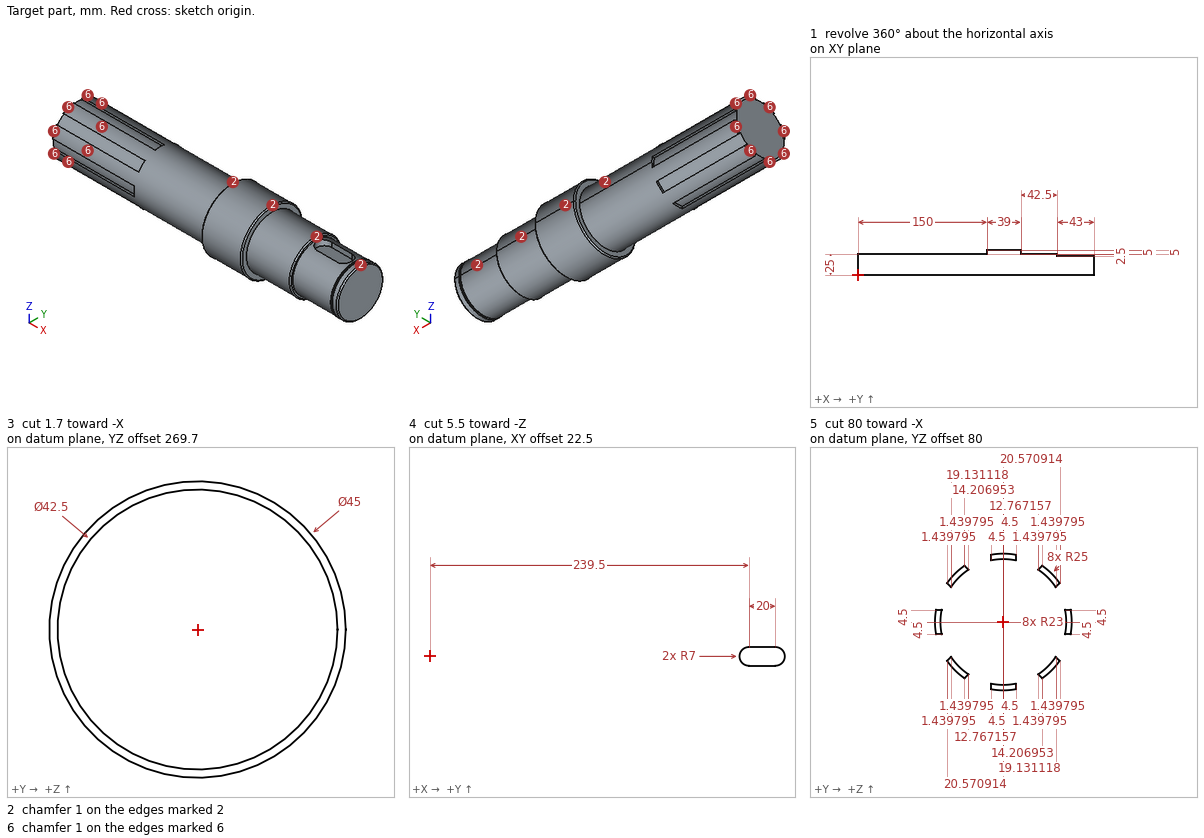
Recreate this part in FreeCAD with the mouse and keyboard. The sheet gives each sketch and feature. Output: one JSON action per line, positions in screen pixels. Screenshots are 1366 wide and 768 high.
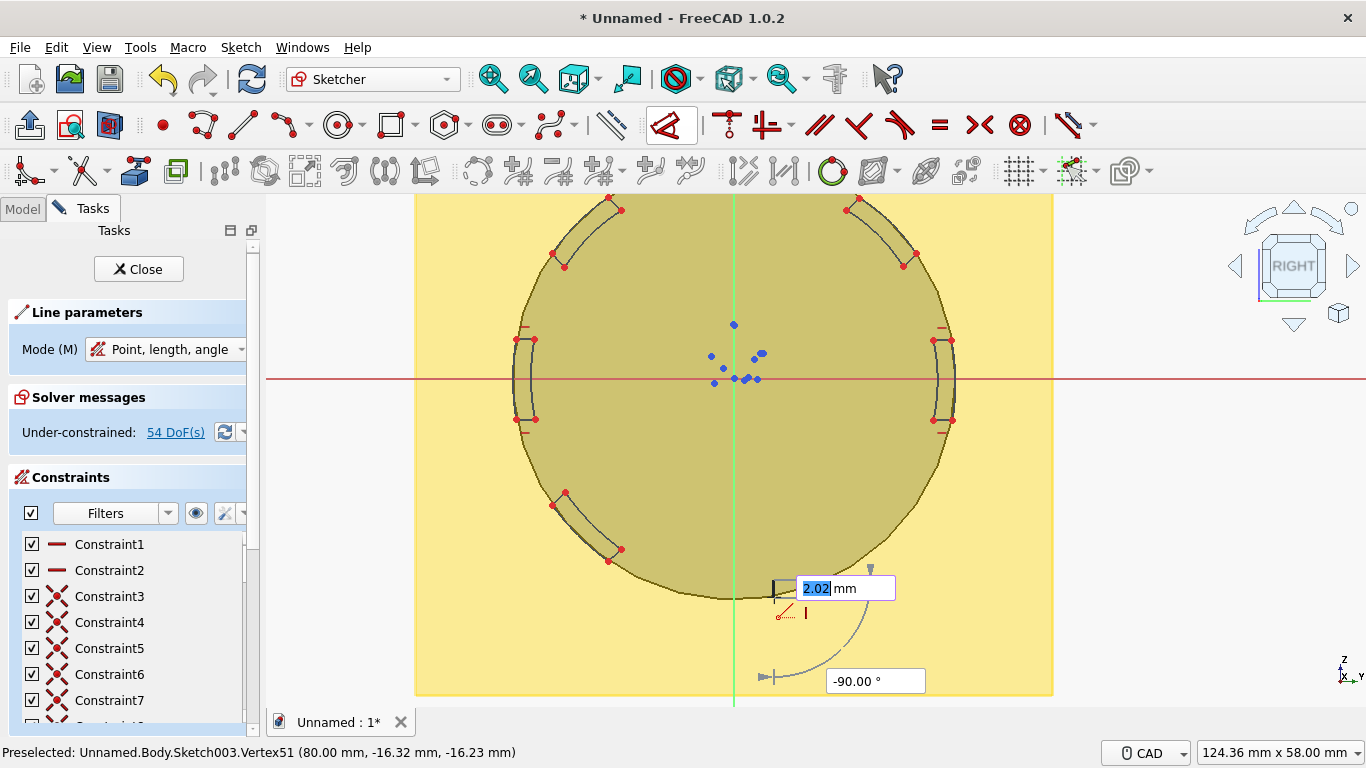
{"action": "left_click", "coordinate": [774, 596]}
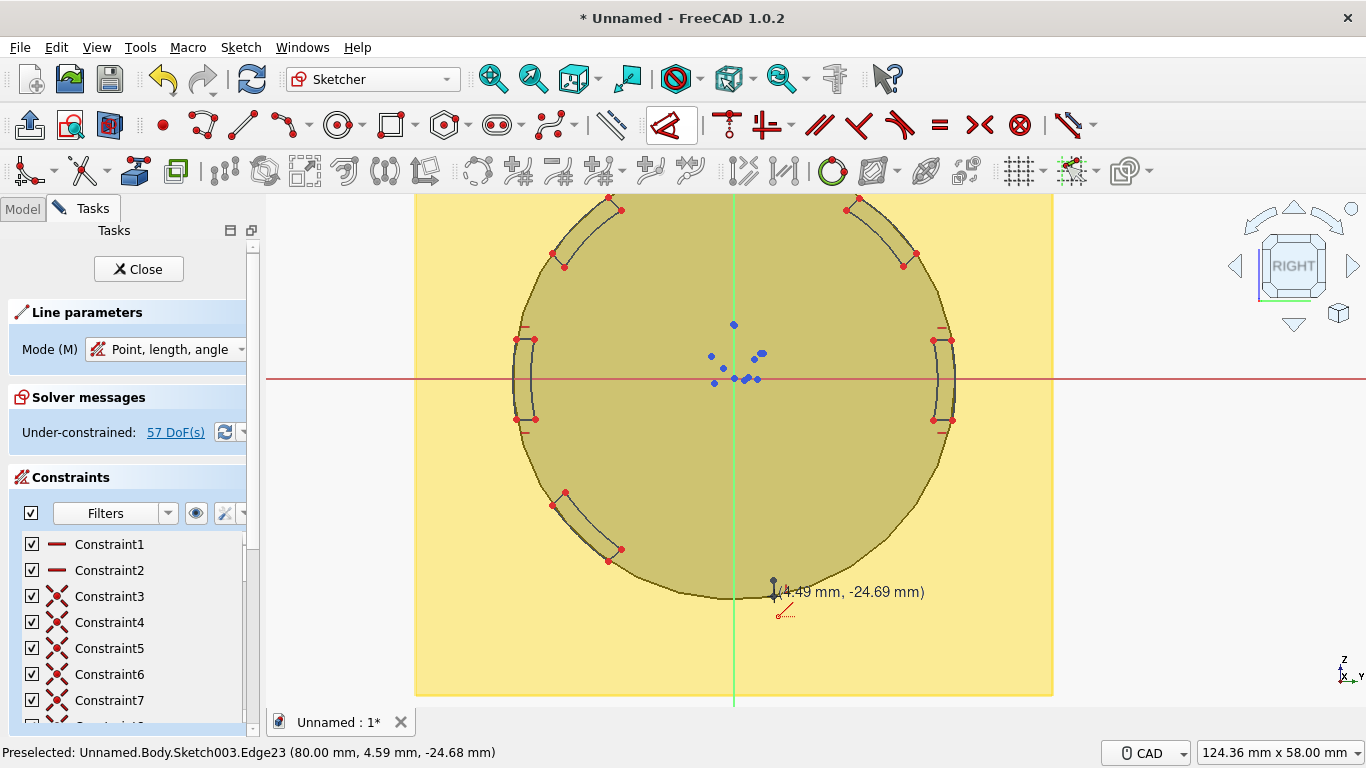
{"action": "left_click", "coordinate": [694, 596]}
{"action": "left_click", "coordinate": [694, 578]}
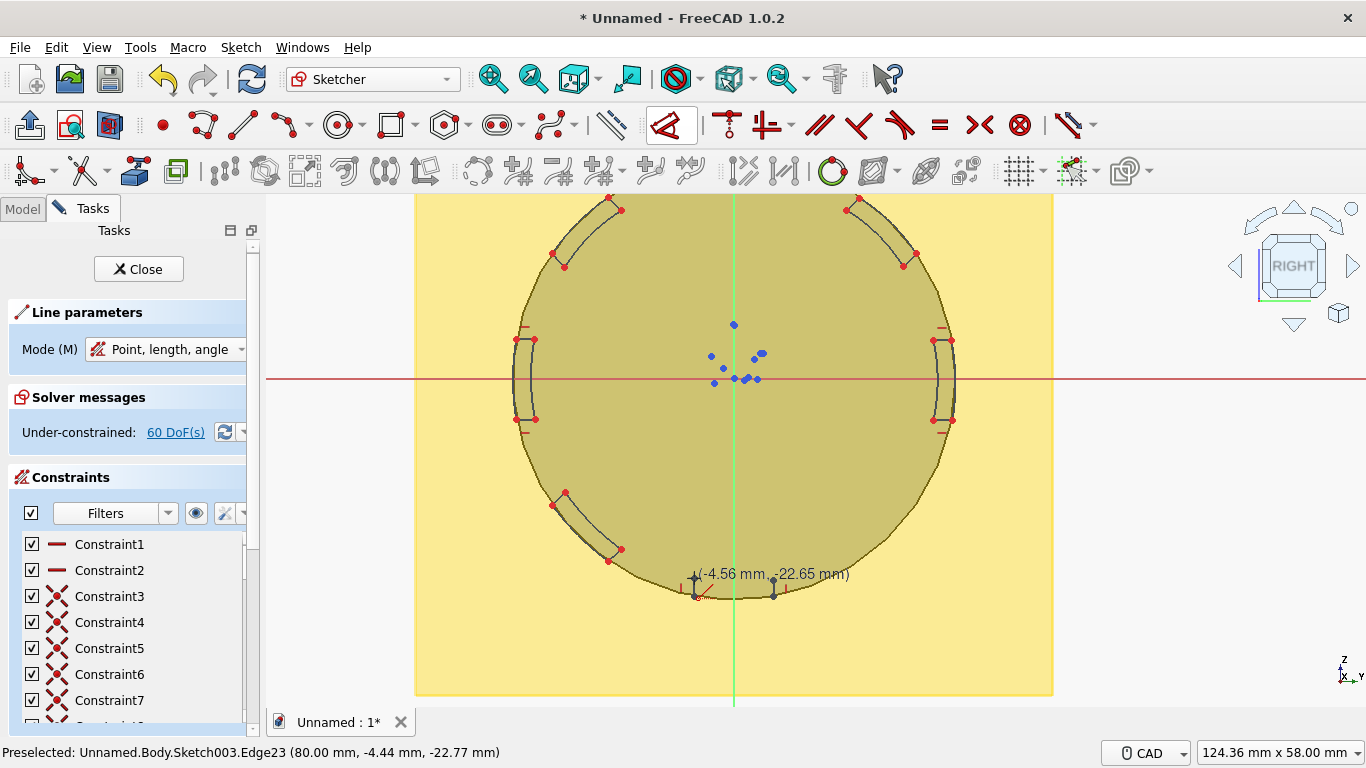
{"action": "left_click", "coordinate": [284, 126]}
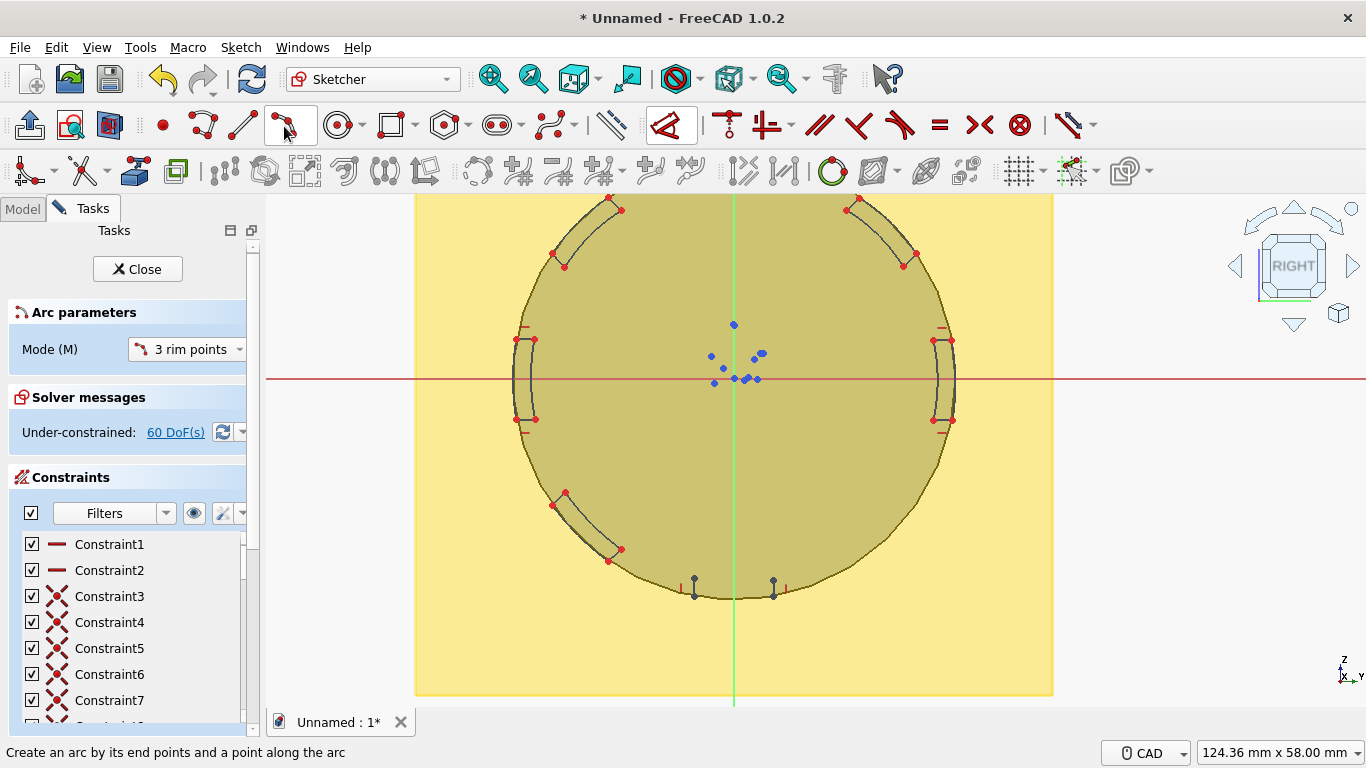
{"action": "scroll", "coordinate": [774, 596], "scroll_direction": "up", "scroll_amount": 3}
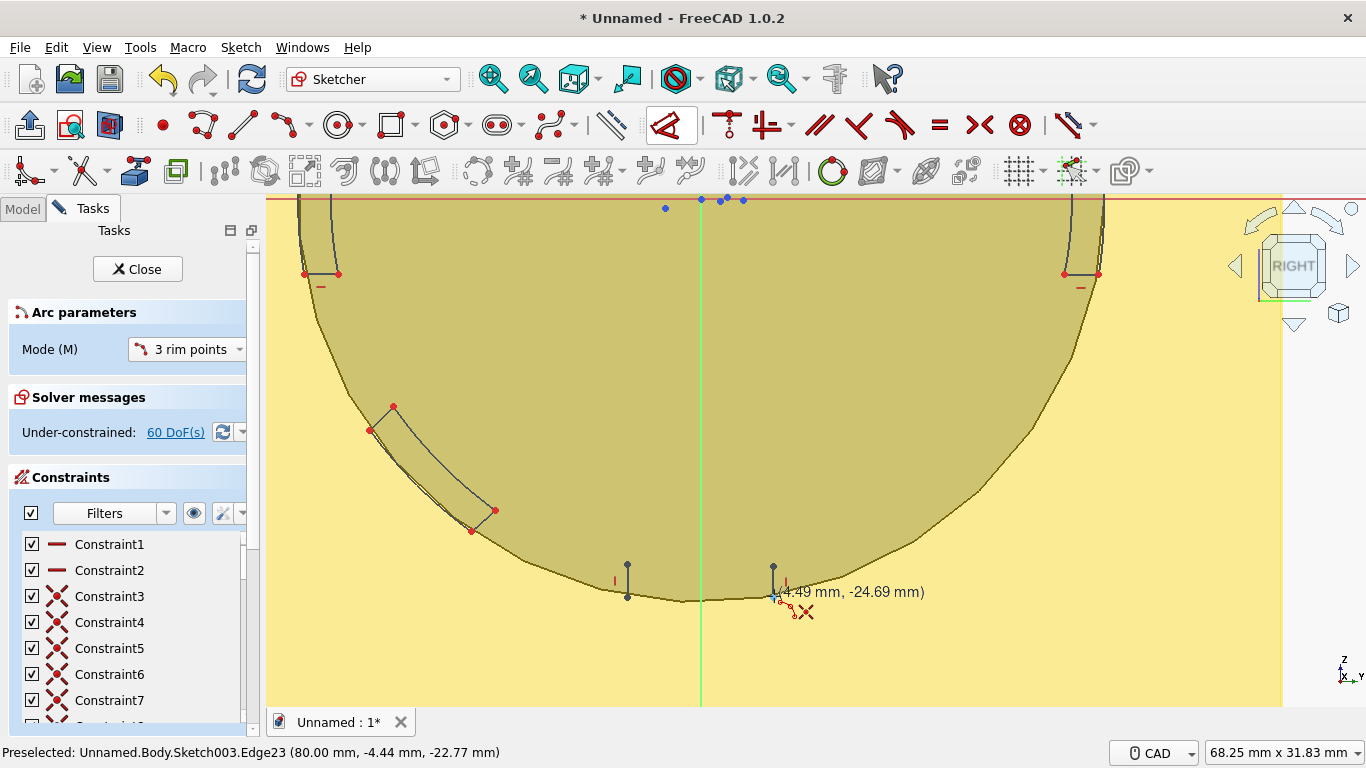
{"action": "left_click", "coordinate": [773, 597]}
{"action": "left_click", "coordinate": [628, 597]}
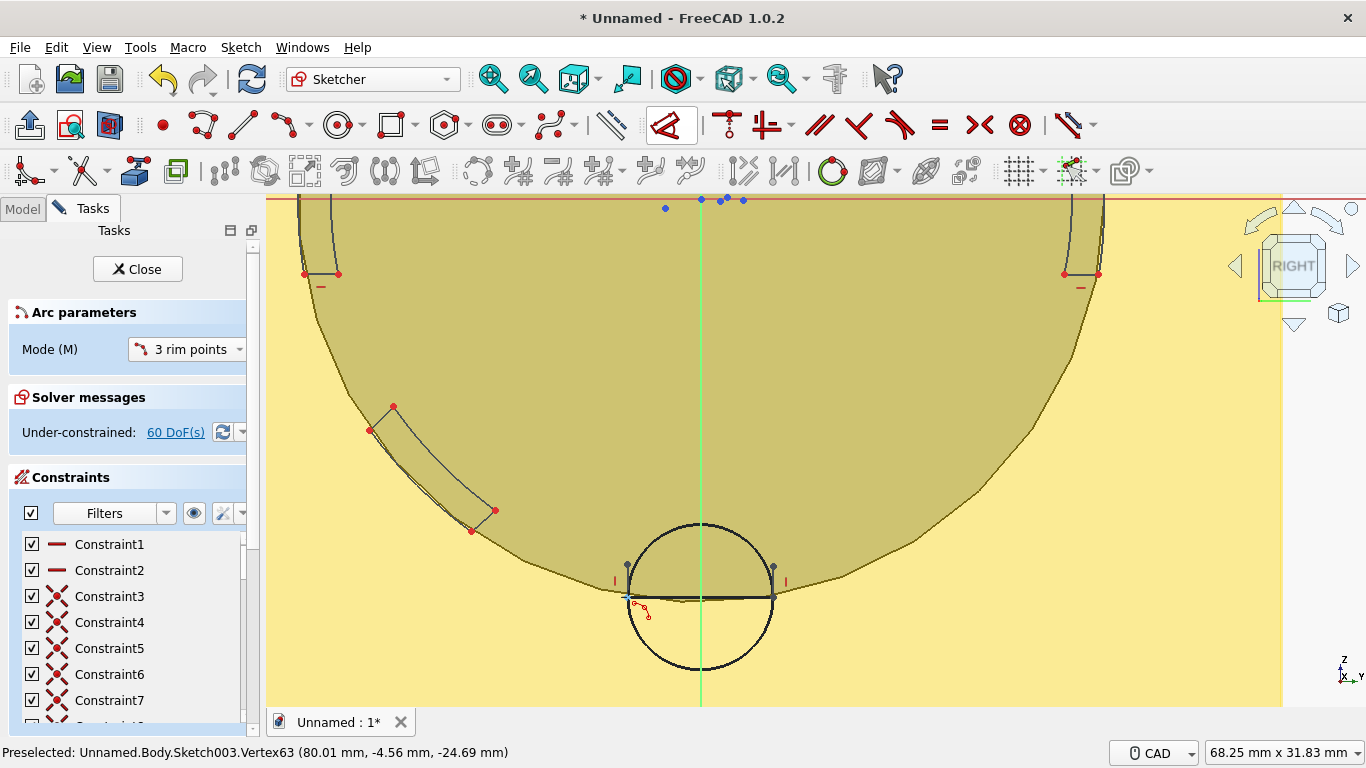
{"action": "scroll", "coordinate": [687, 602], "scroll_direction": "up", "scroll_amount": 5}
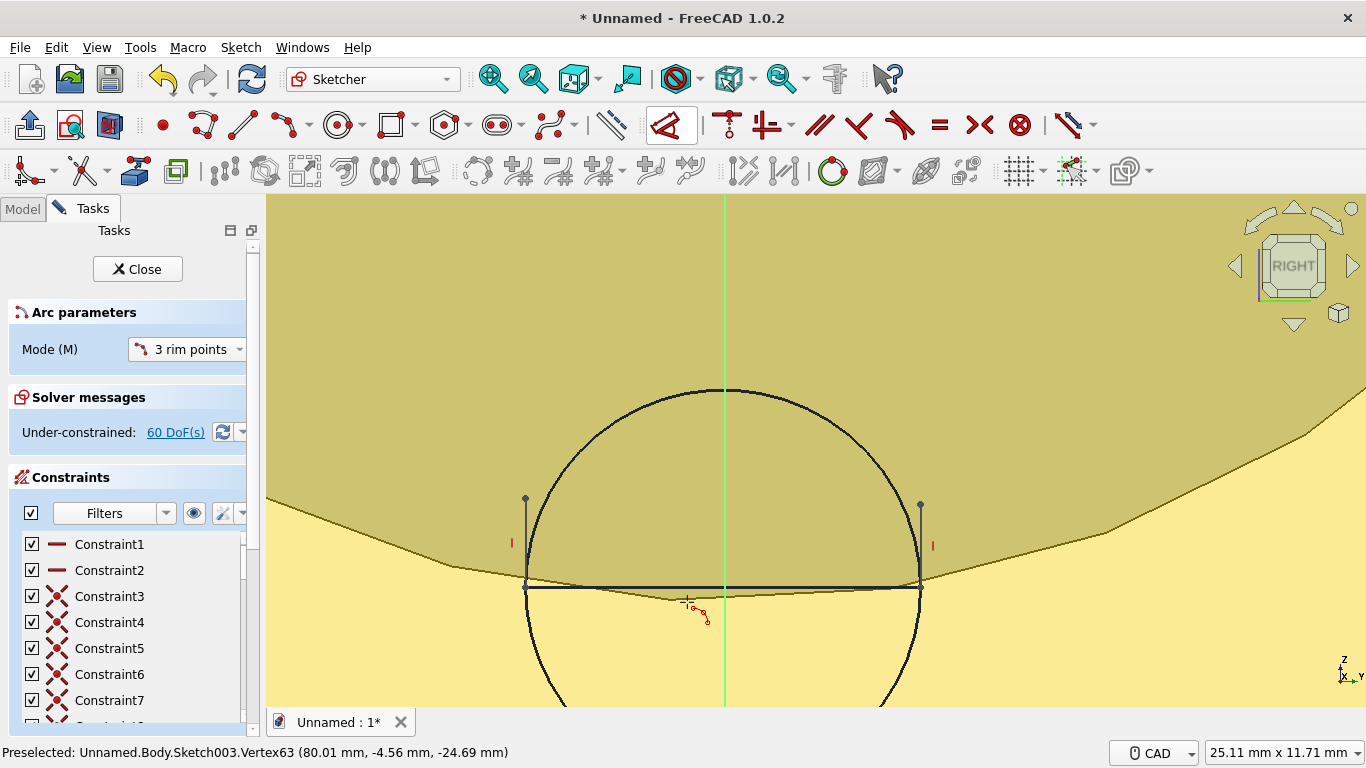
{"action": "left_click", "coordinate": [686, 601]}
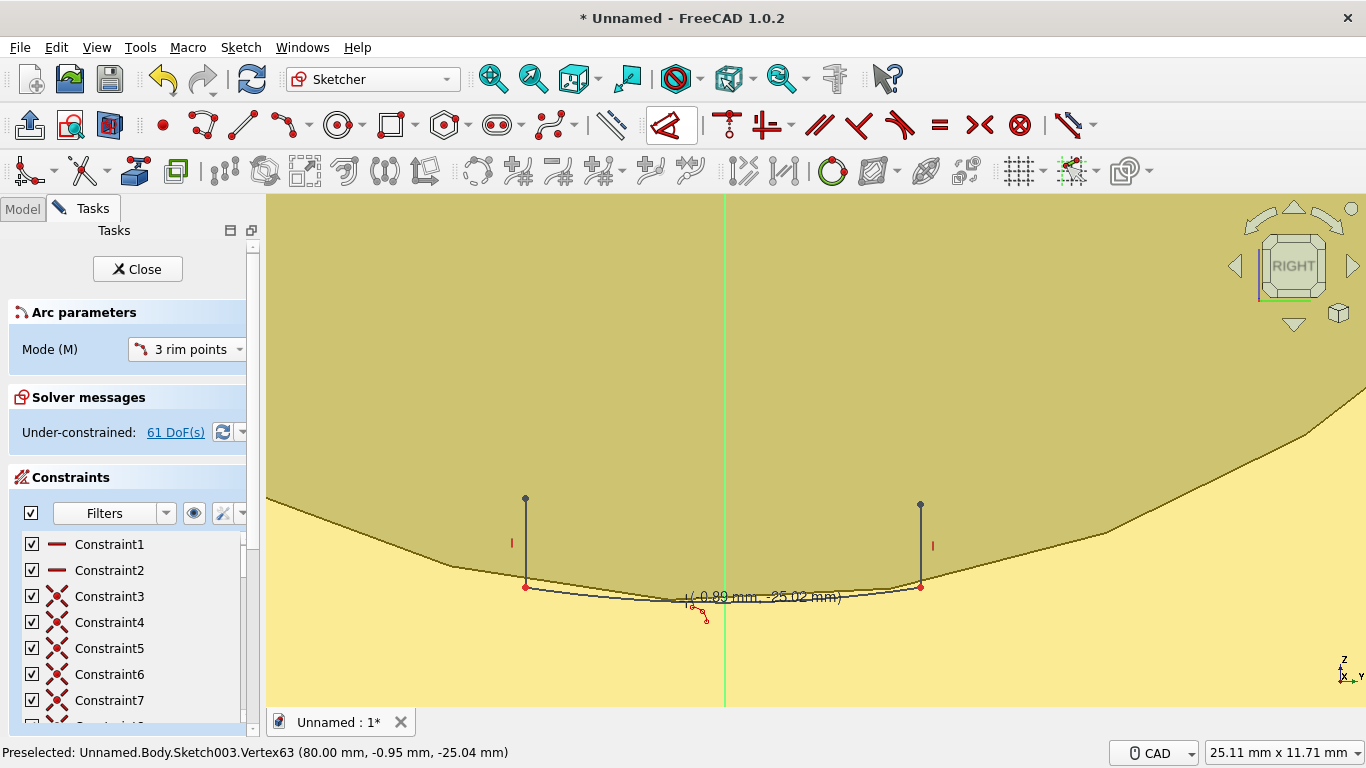
{"action": "left_click", "coordinate": [526, 498]}
{"action": "left_click", "coordinate": [921, 504]}
{"action": "left_click", "coordinate": [685, 513]}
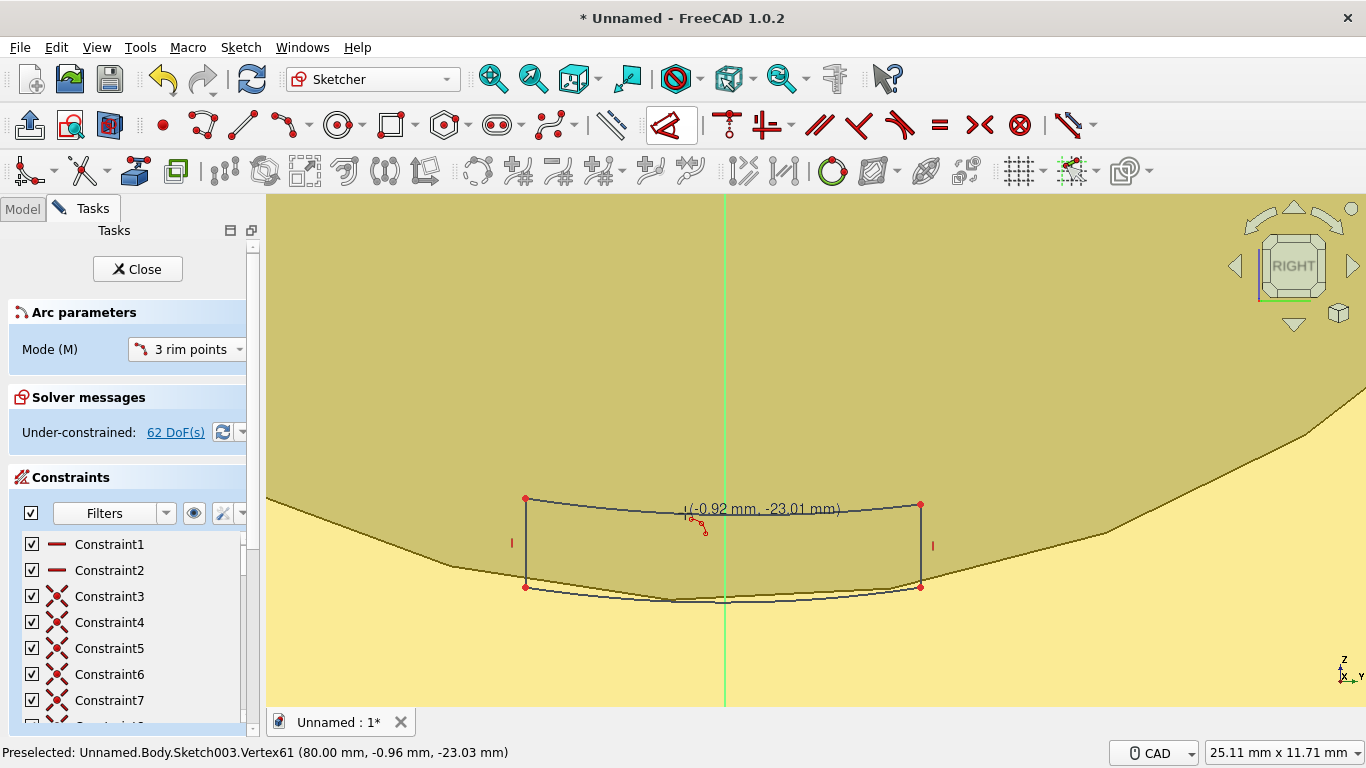
{"action": "left_click", "coordinate": [244, 126]}